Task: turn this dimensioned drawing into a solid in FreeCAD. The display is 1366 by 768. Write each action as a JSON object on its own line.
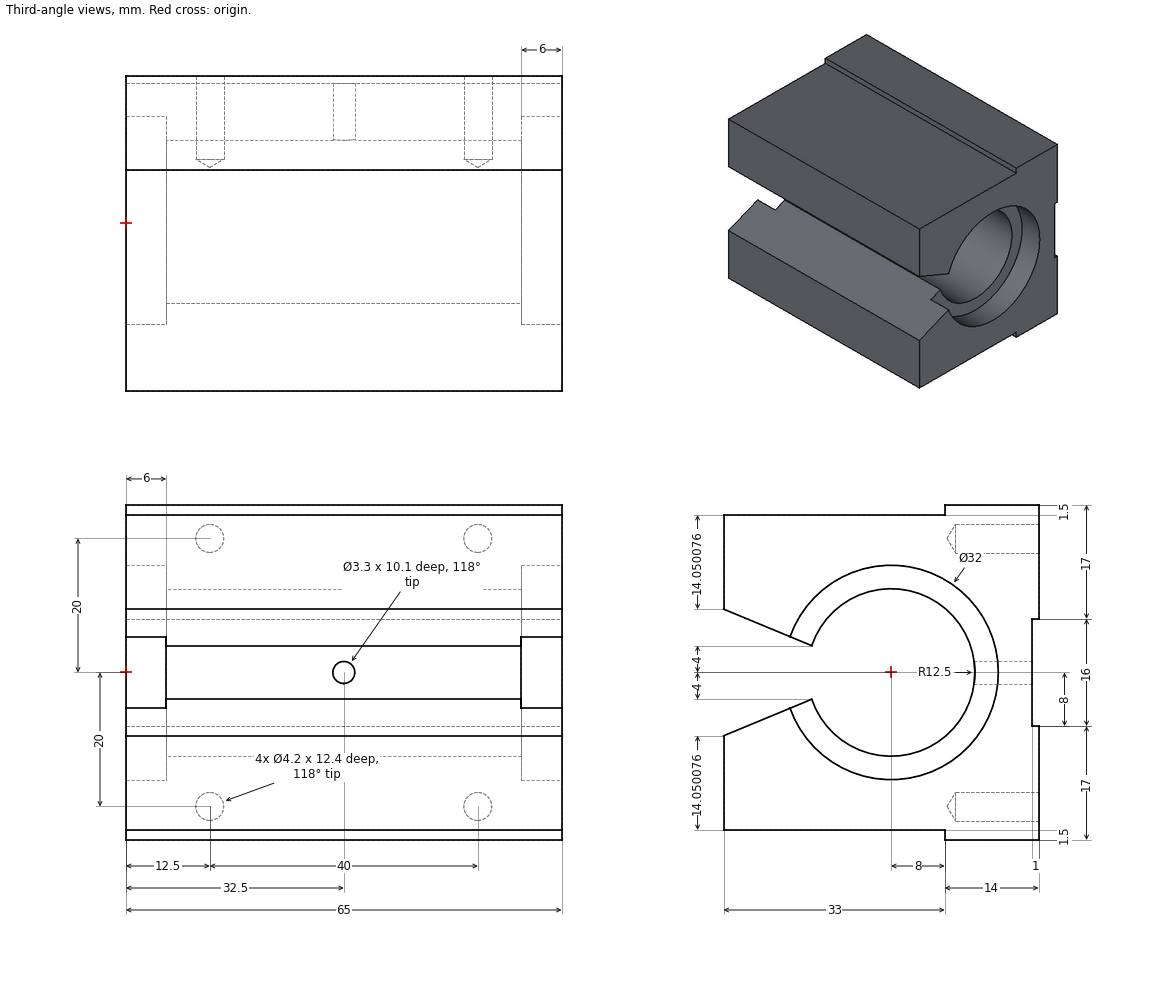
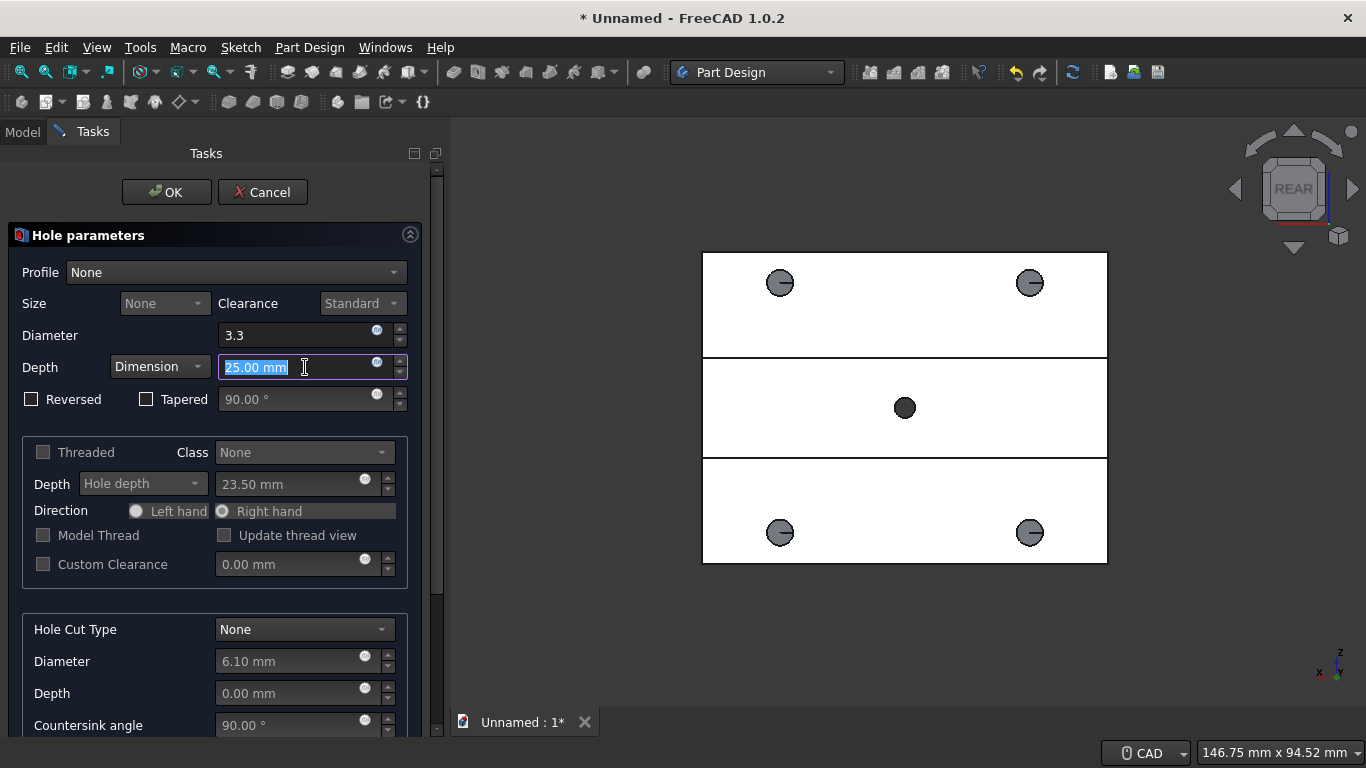
{"action": "type", "text": "10.1"}
{"action": "key", "text": "Tab"}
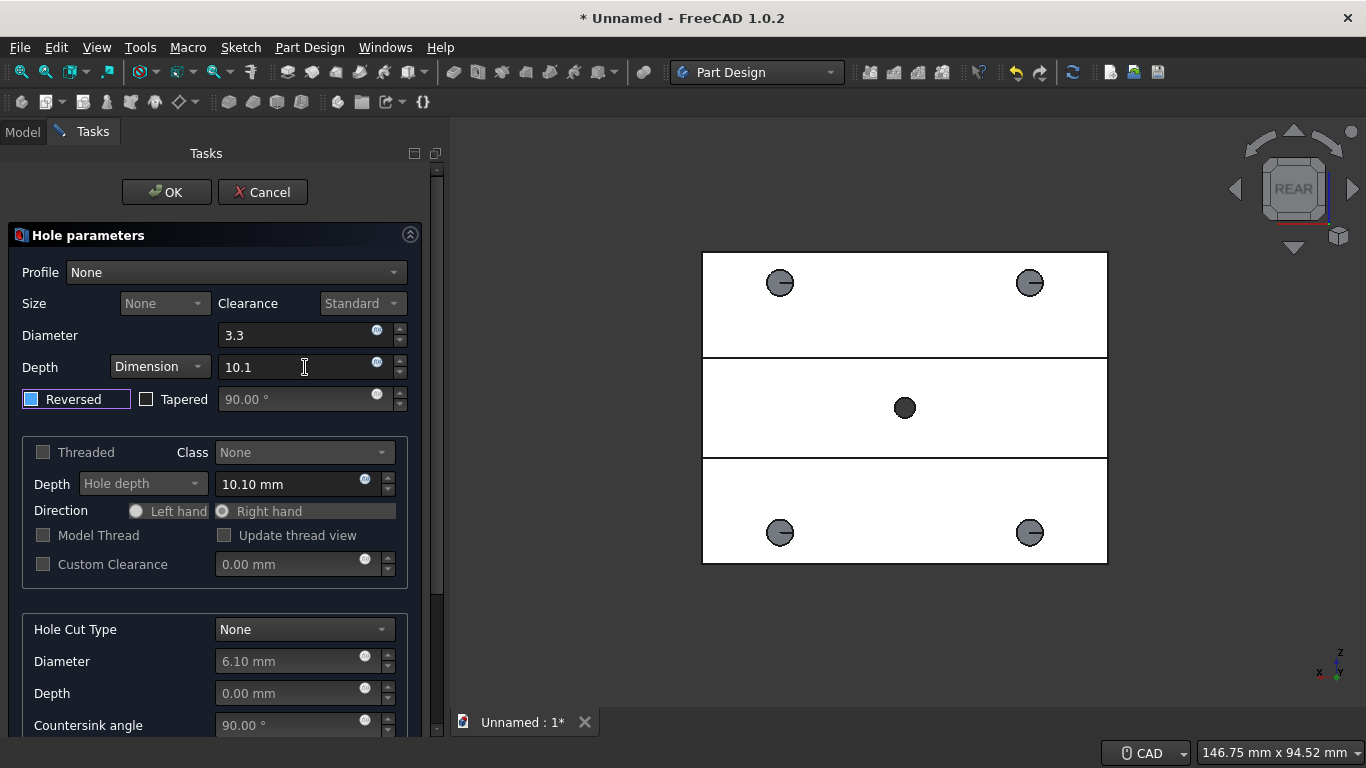
{"action": "left_click", "coordinate": [167, 192]}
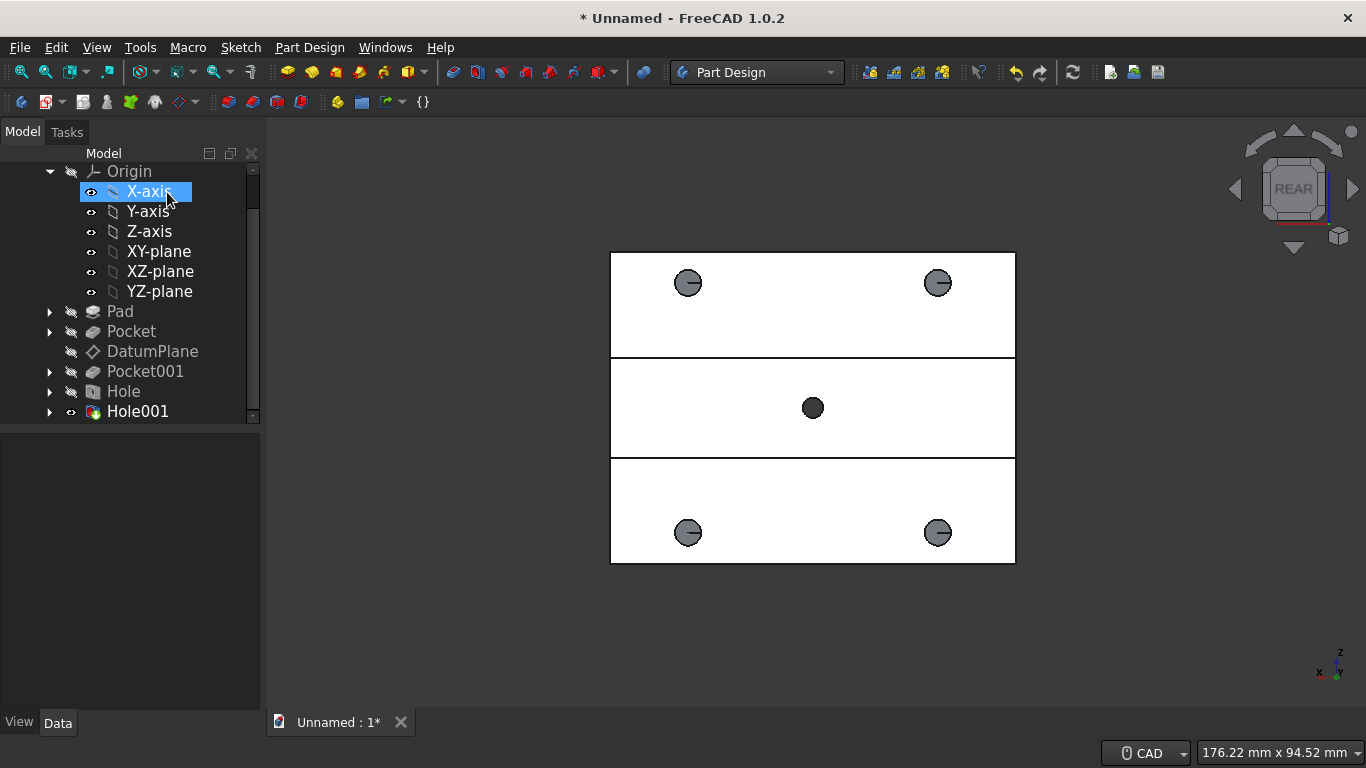
{"action": "key", "text": "0"}